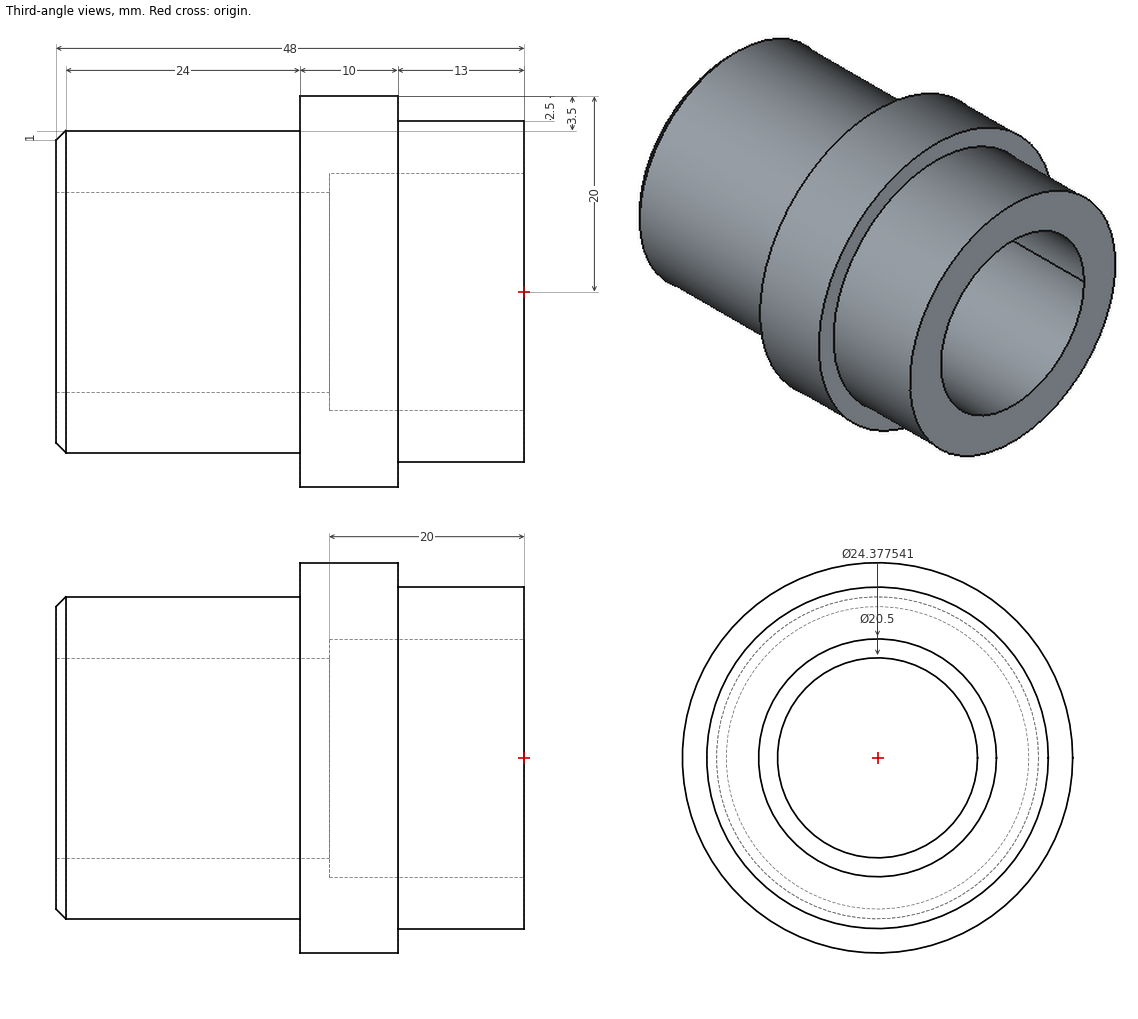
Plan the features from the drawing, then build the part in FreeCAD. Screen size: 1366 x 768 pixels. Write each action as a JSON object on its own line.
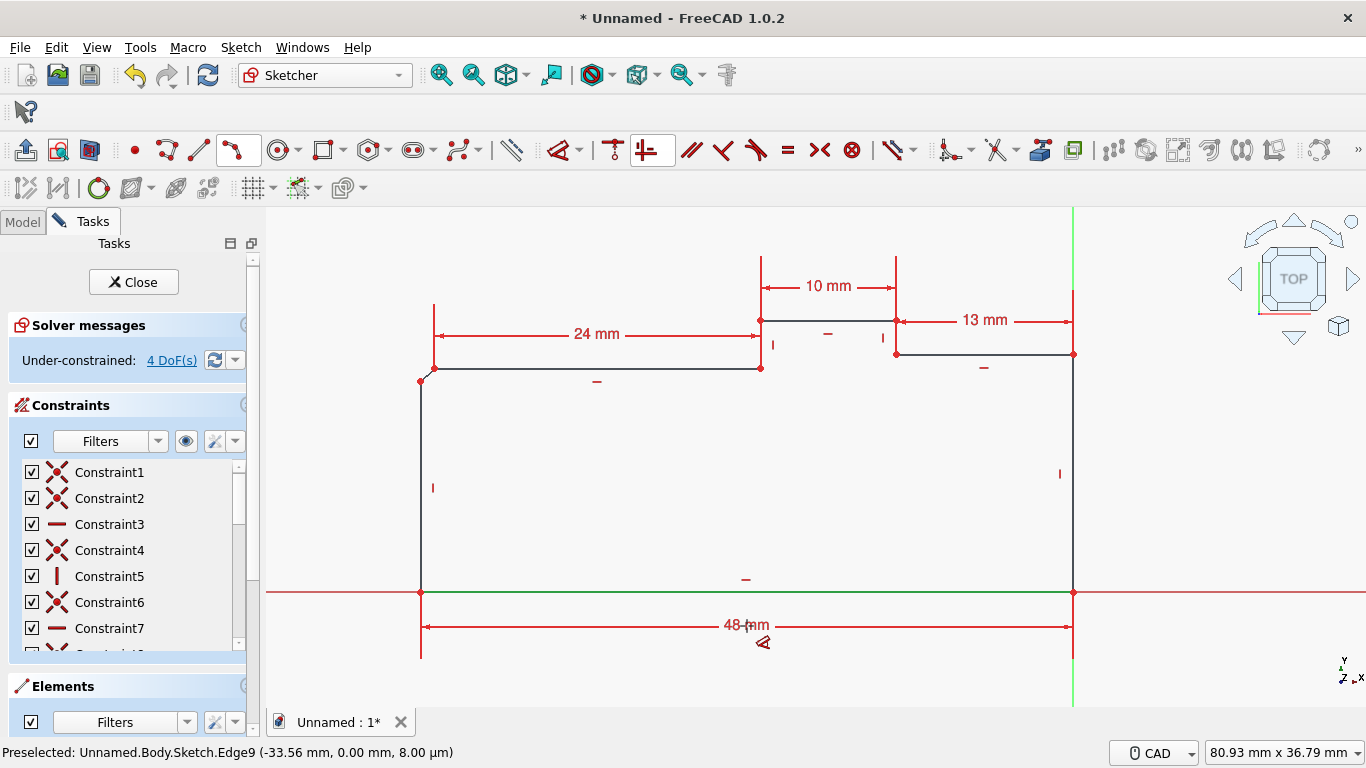
{"action": "scroll", "coordinate": [428, 376], "scroll_direction": "up", "scroll_amount": 6}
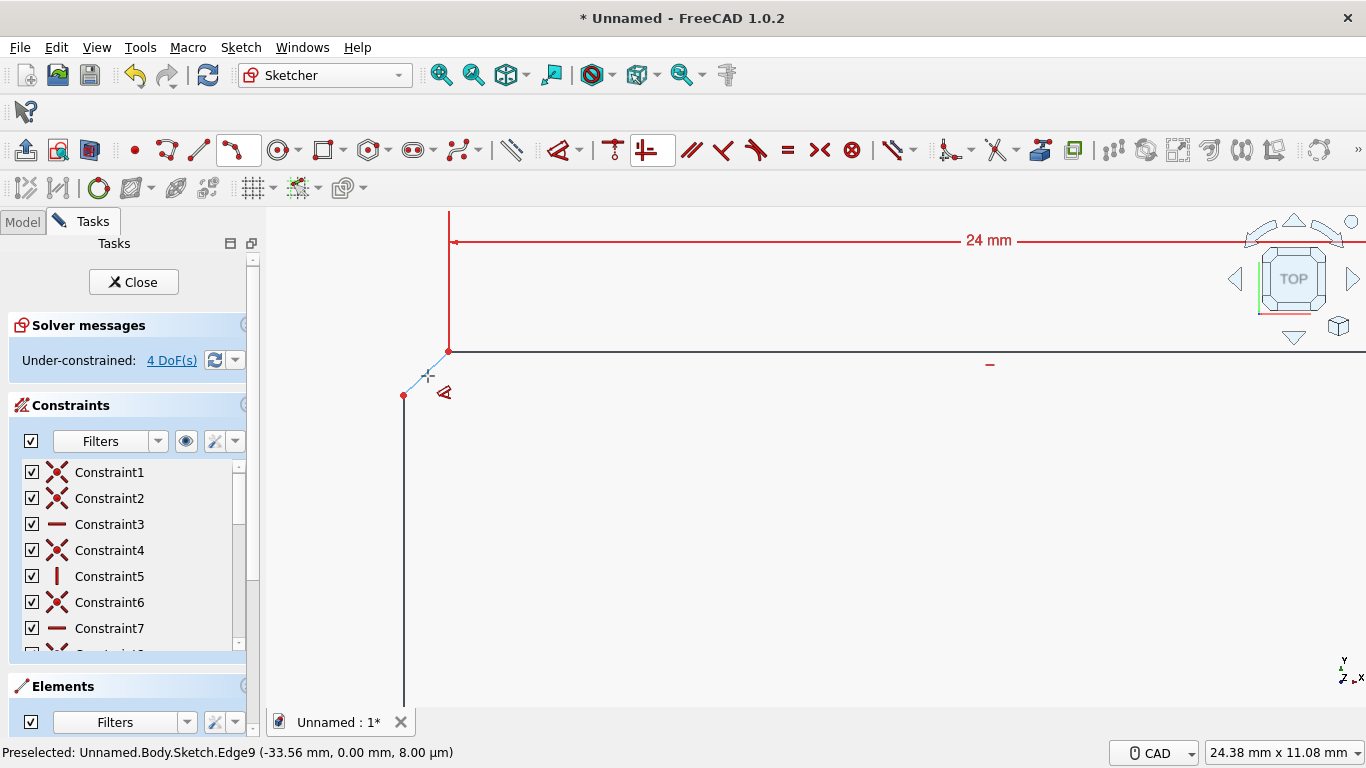
{"action": "left_click", "coordinate": [426, 374]}
{"action": "left_click", "coordinate": [370, 374]}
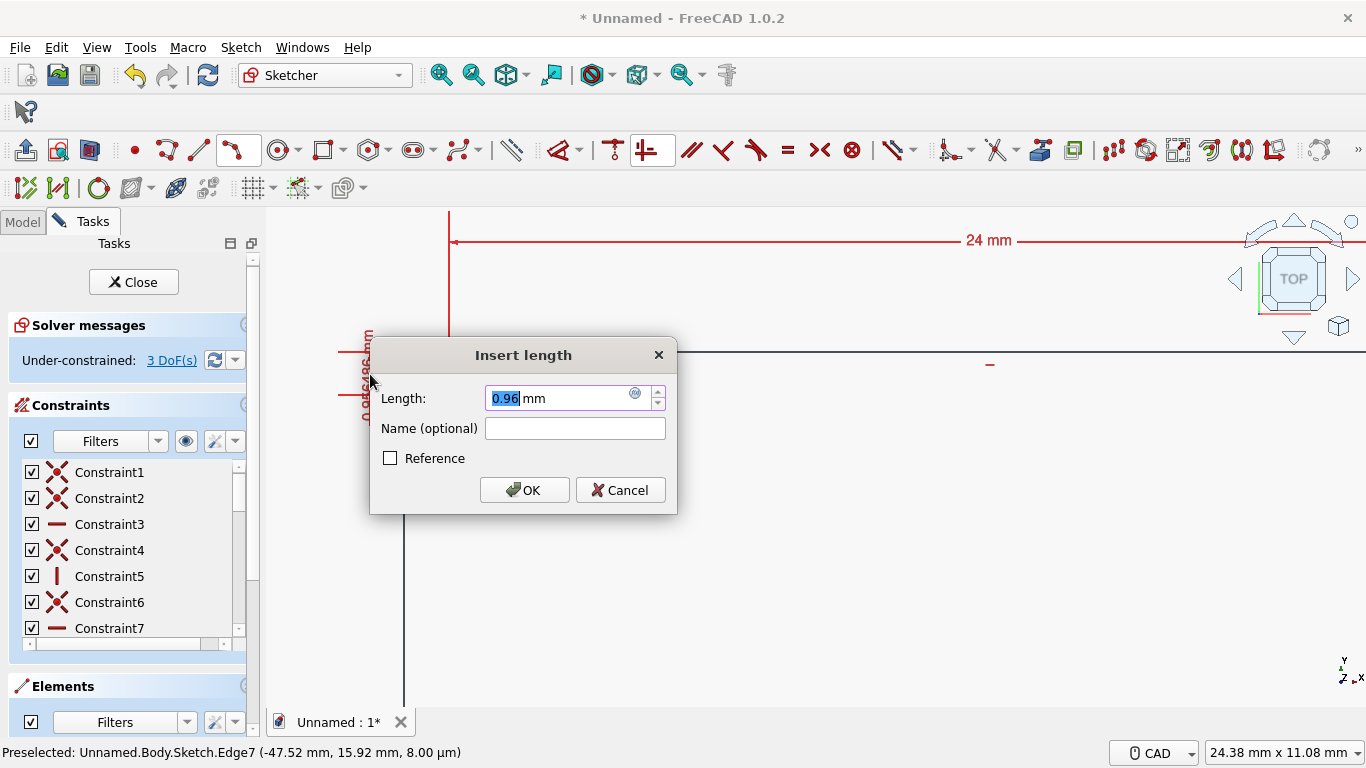
{"action": "type", "text": "1"}
{"action": "key", "text": "Return"}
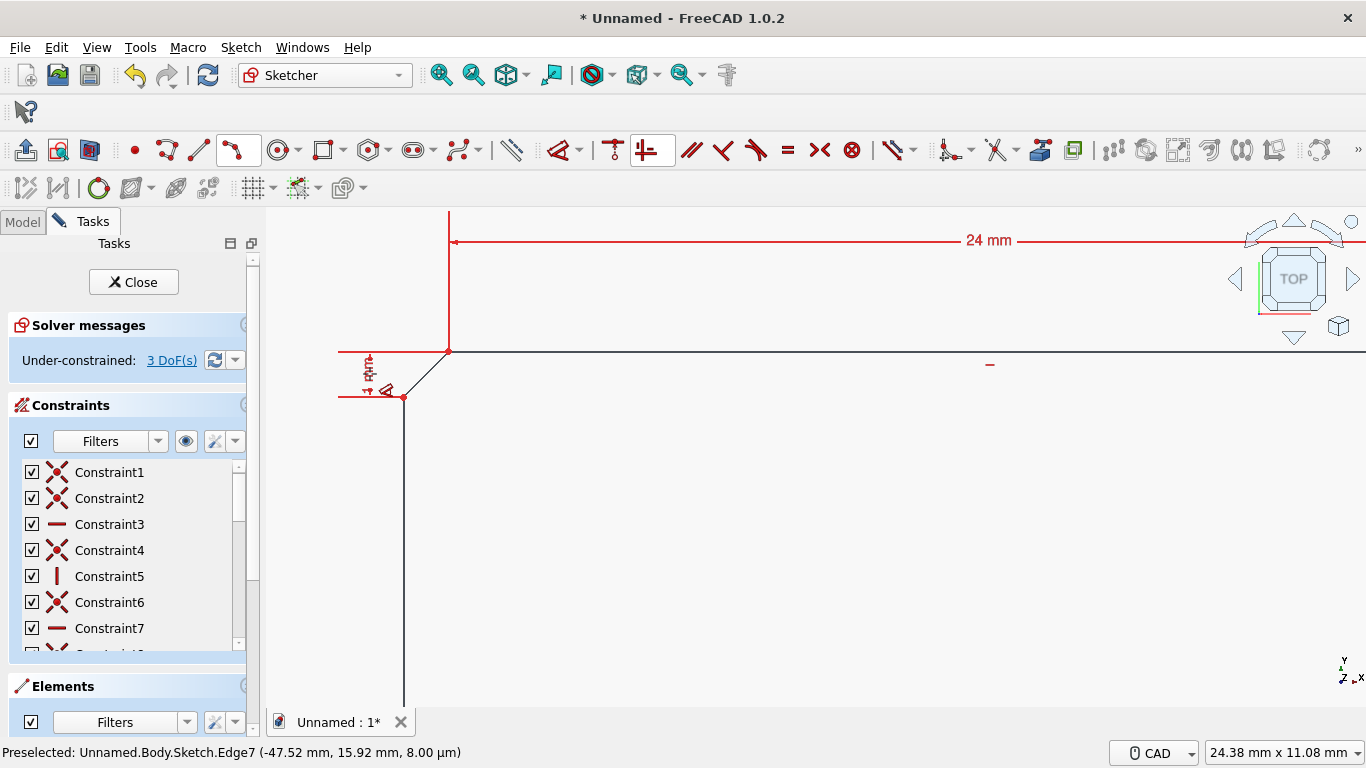
{"action": "scroll", "coordinate": [429, 377], "scroll_direction": "down", "scroll_amount": 6}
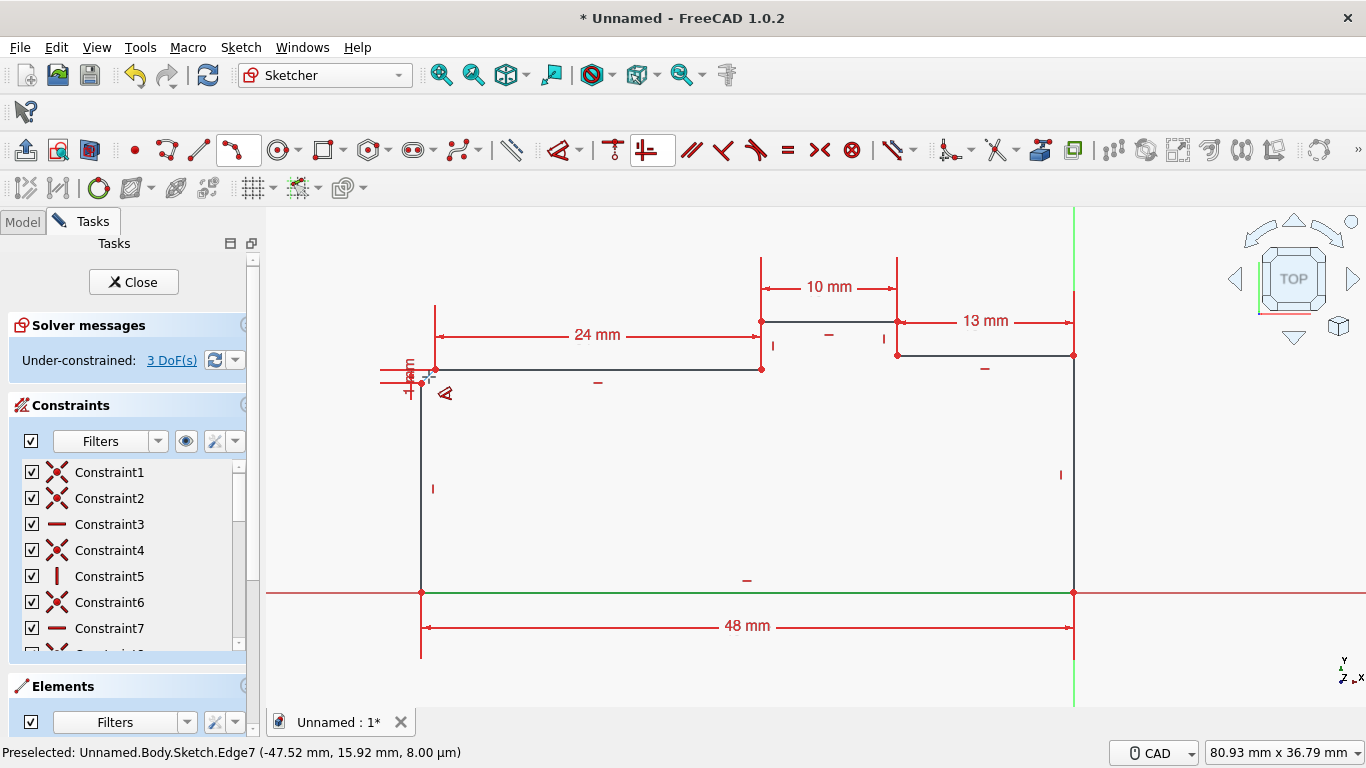
{"action": "scroll", "coordinate": [897, 346], "scroll_direction": "up", "scroll_amount": 2}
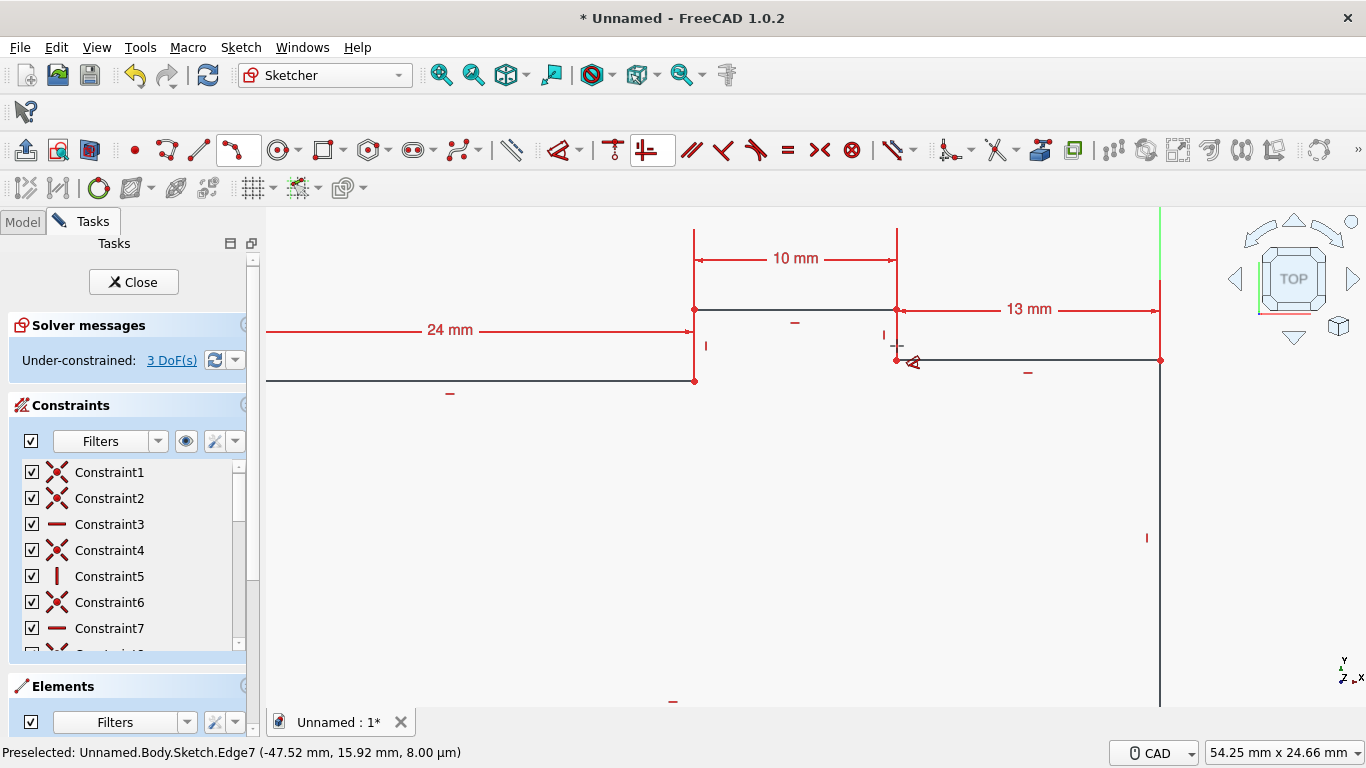
{"action": "left_click", "coordinate": [897, 345]}
{"action": "left_click", "coordinate": [931, 335]}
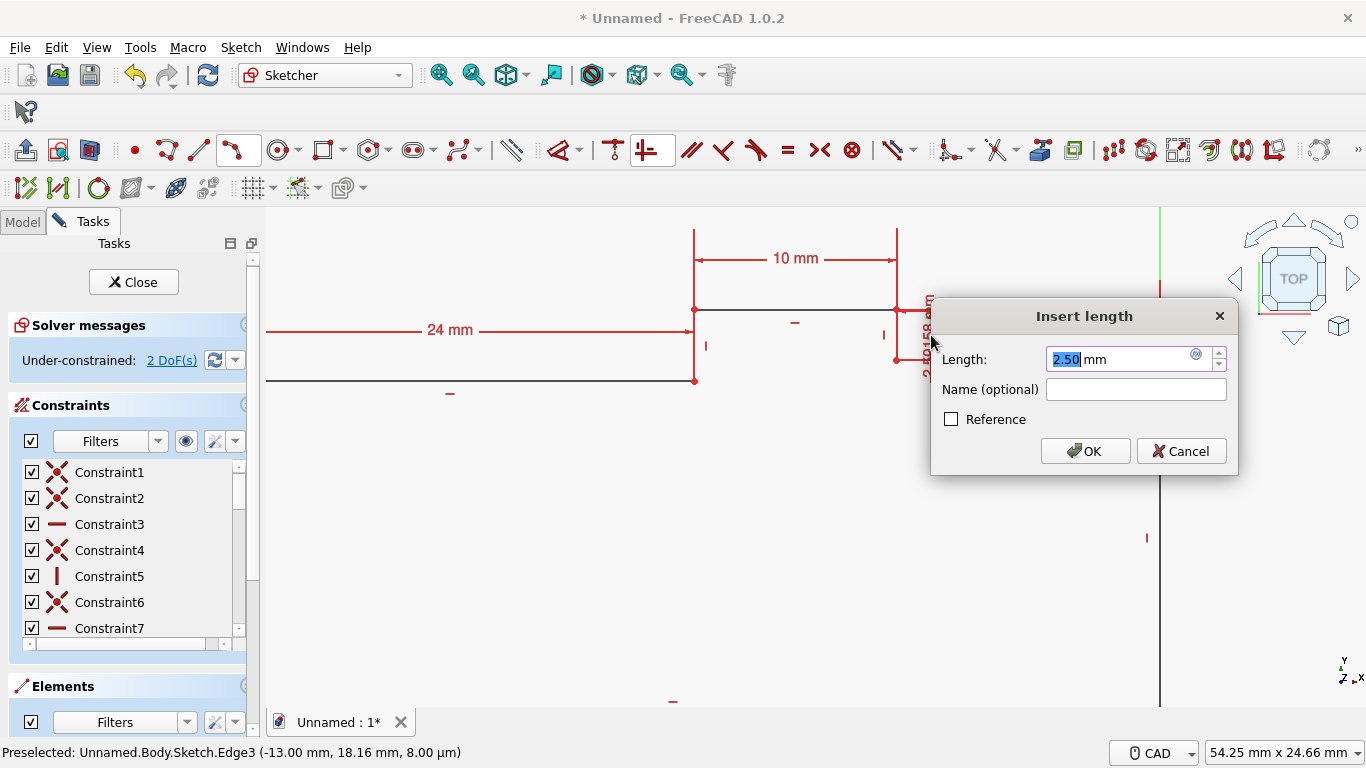
{"action": "type", "text": "2.5"}
{"action": "key", "text": "Return"}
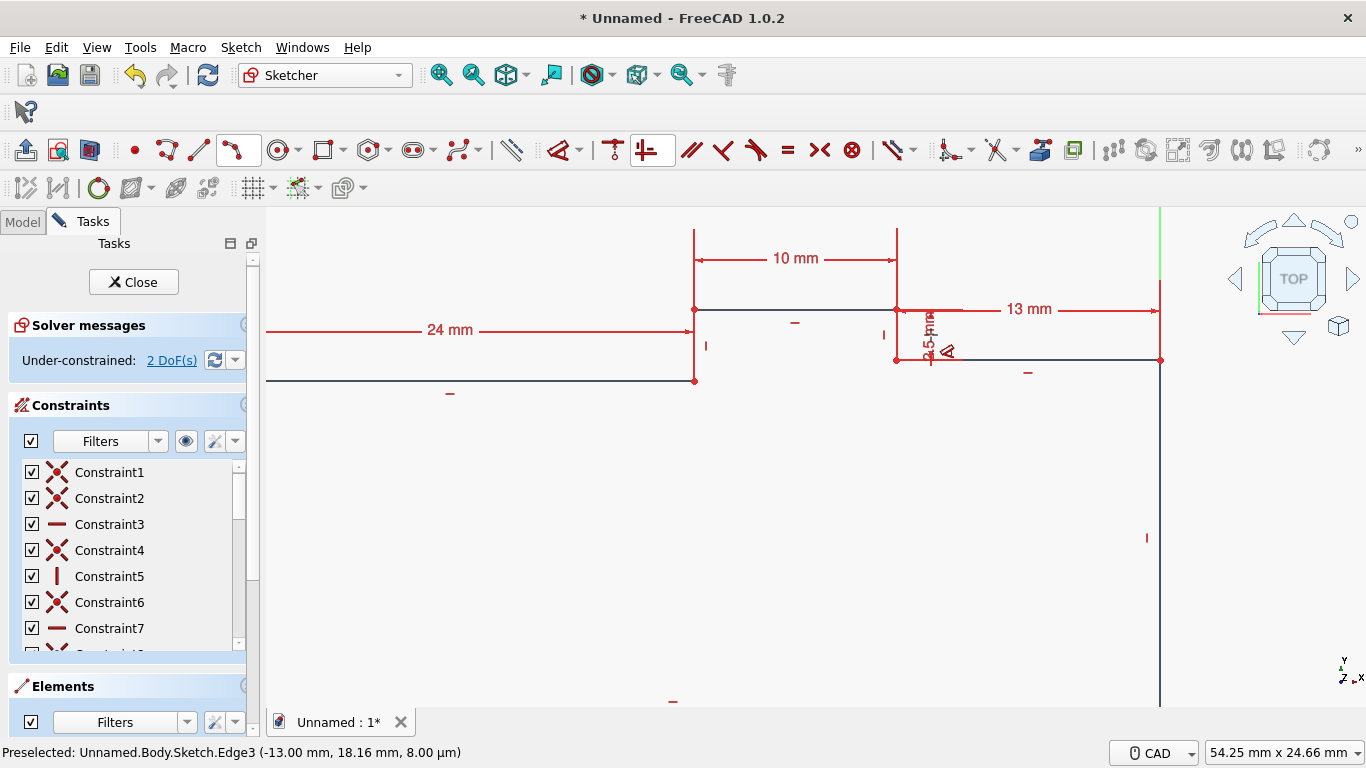
{"action": "left_click", "coordinate": [694, 331]}
{"action": "left_click", "coordinate": [728, 345]}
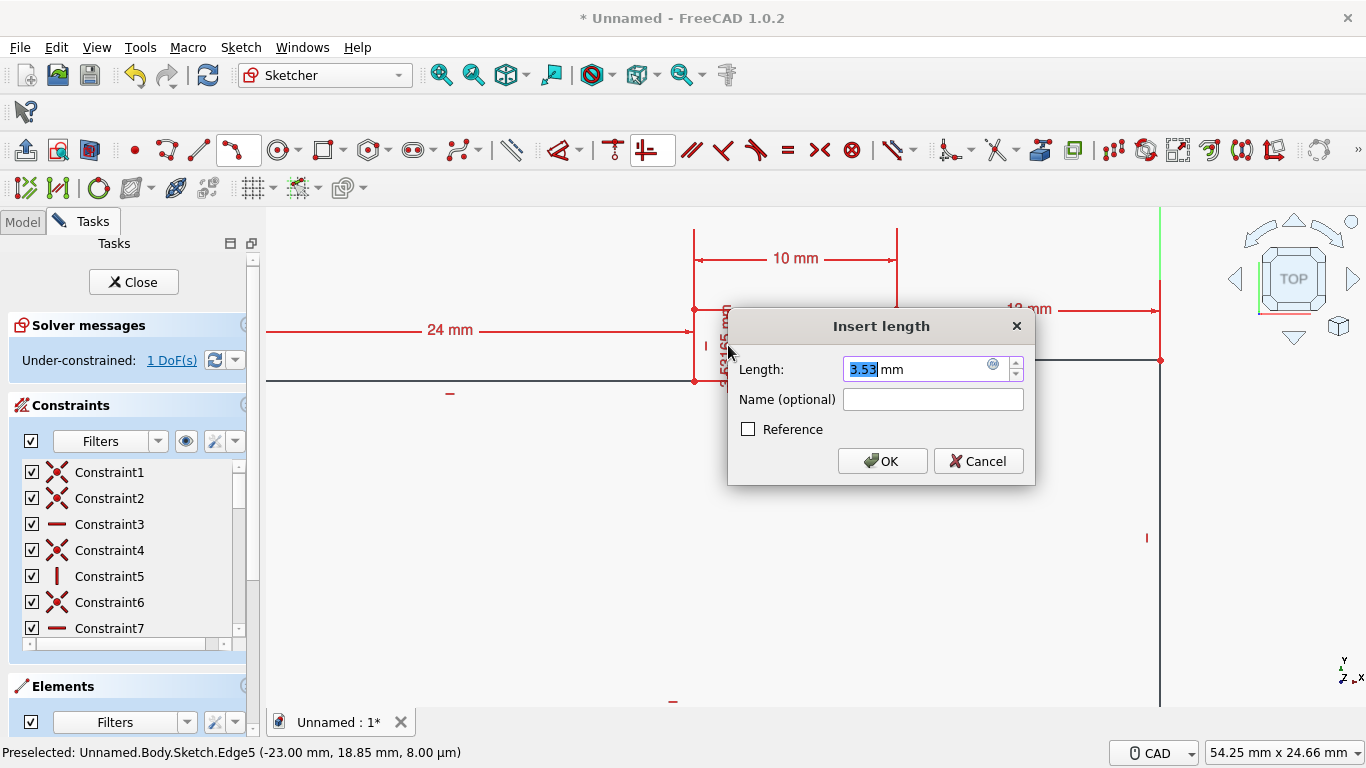
{"action": "type", "text": "3.5"}
{"action": "key", "text": "Return"}